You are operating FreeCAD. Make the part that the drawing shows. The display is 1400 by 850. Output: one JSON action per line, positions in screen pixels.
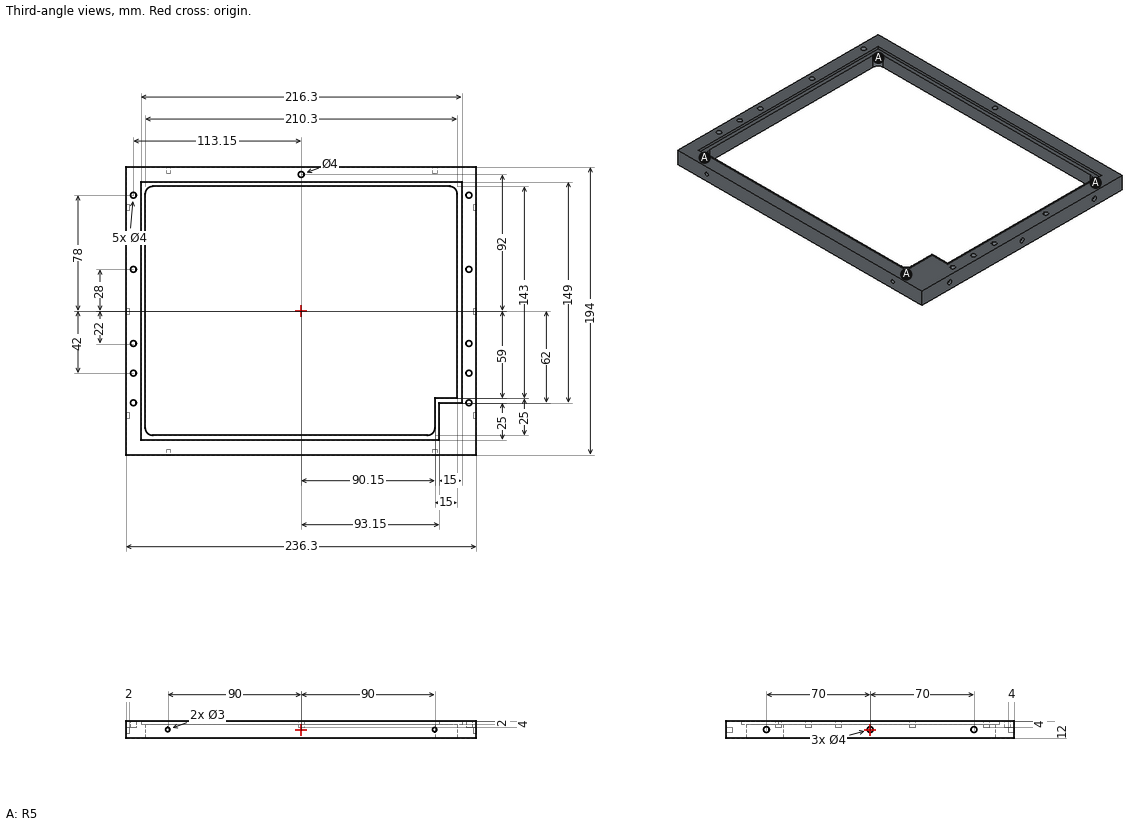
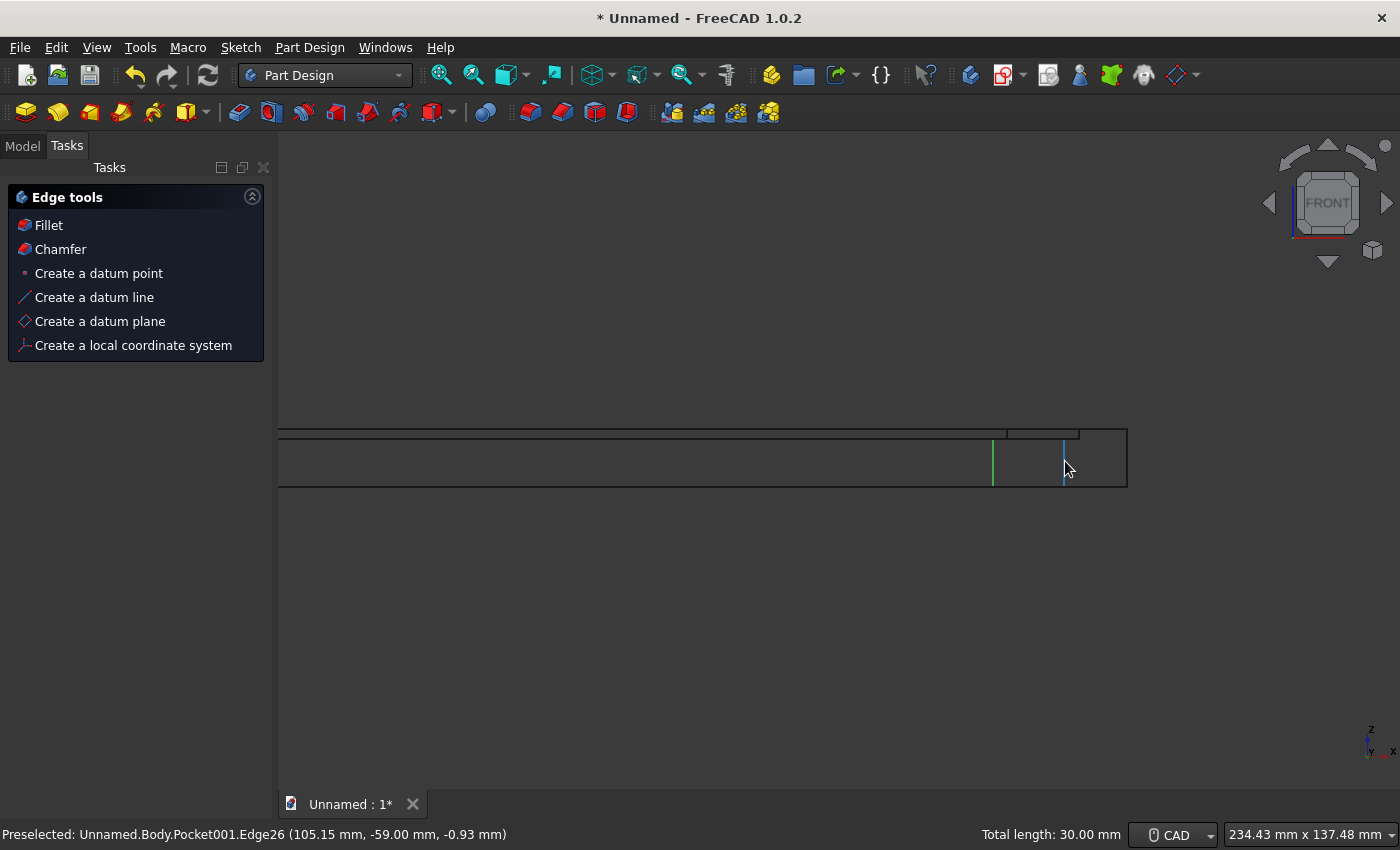
{"action": "left_click", "coordinate": [442, 76]}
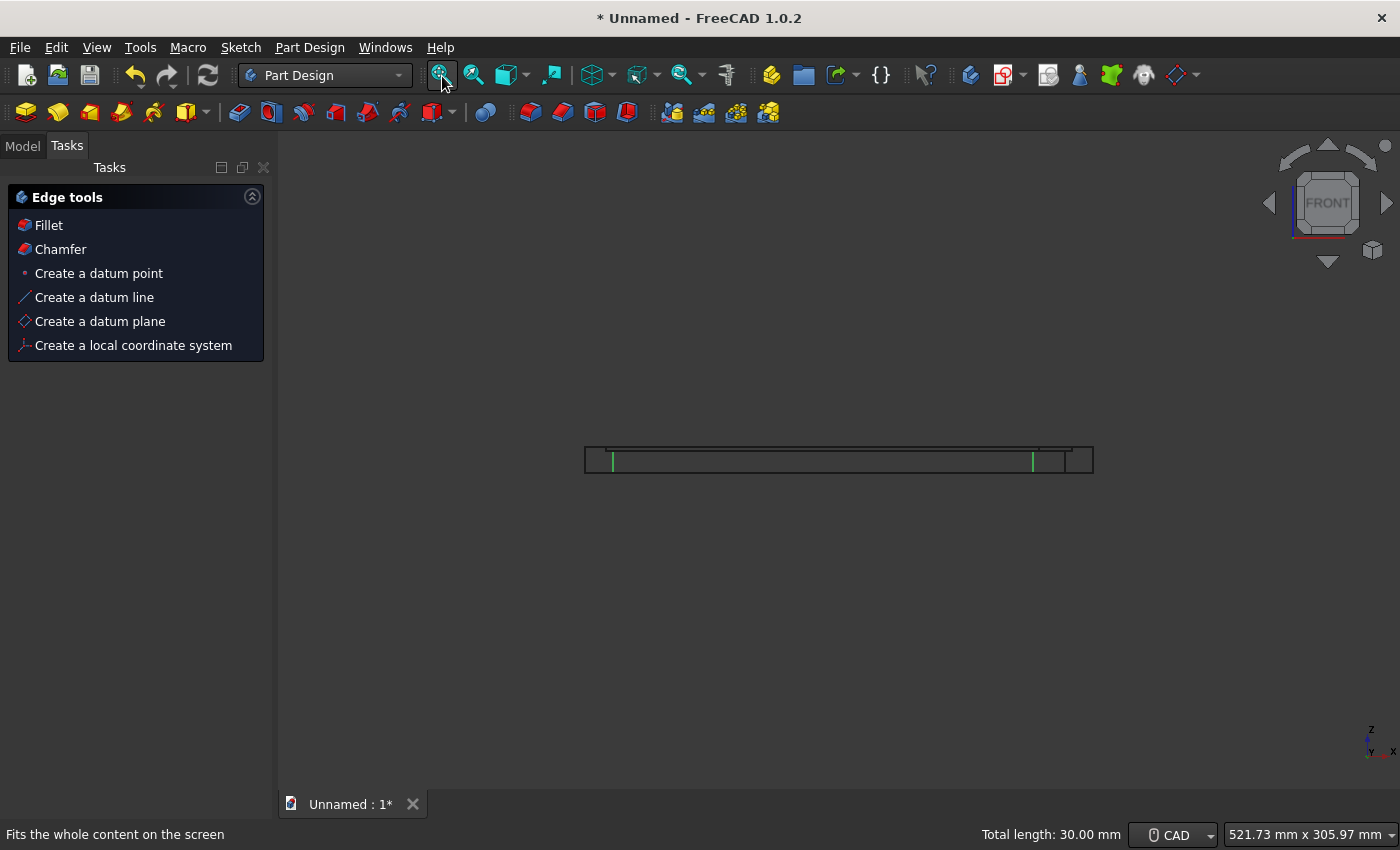
{"action": "key", "text": "3"}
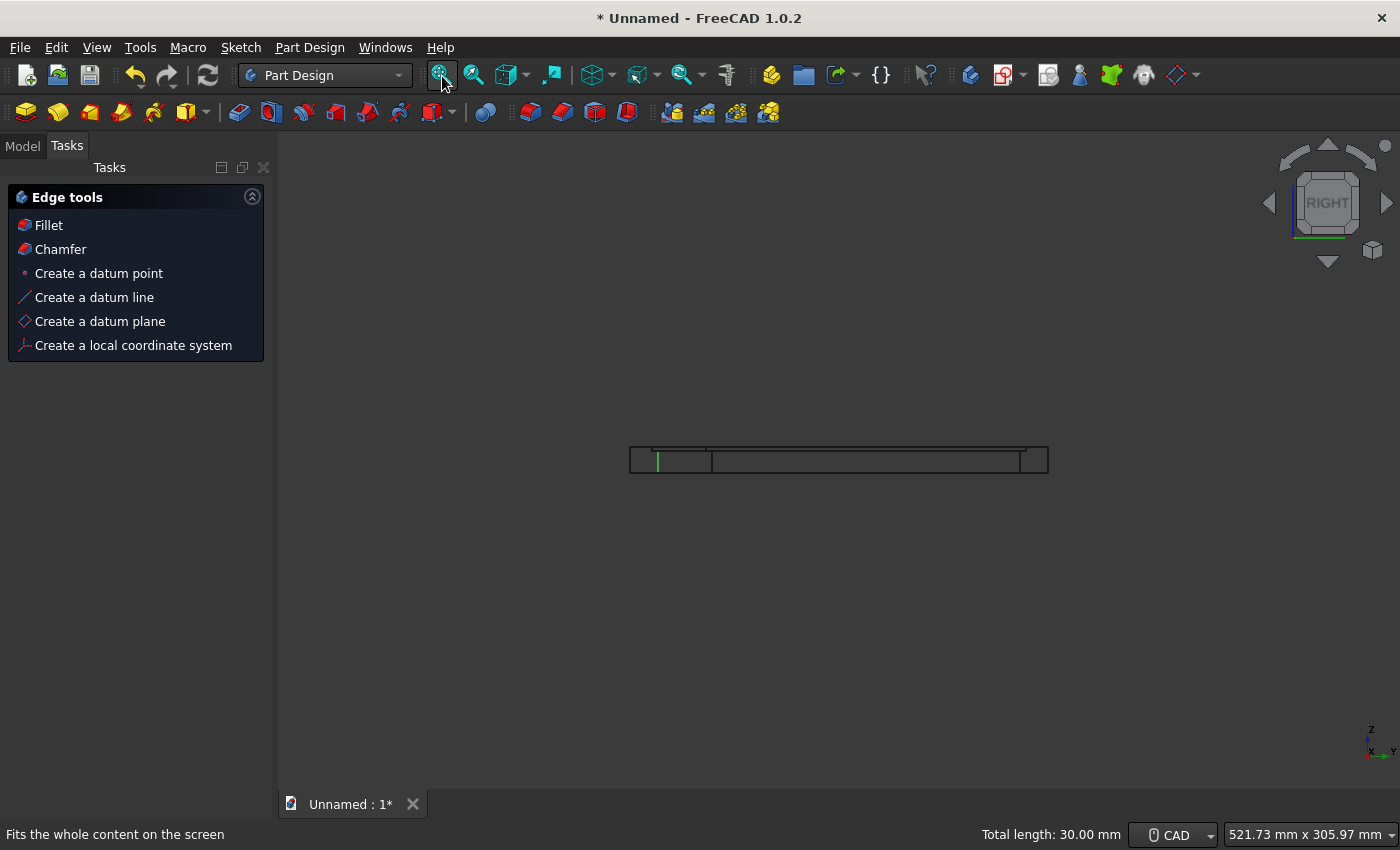
{"action": "left_click", "coordinate": [442, 76]}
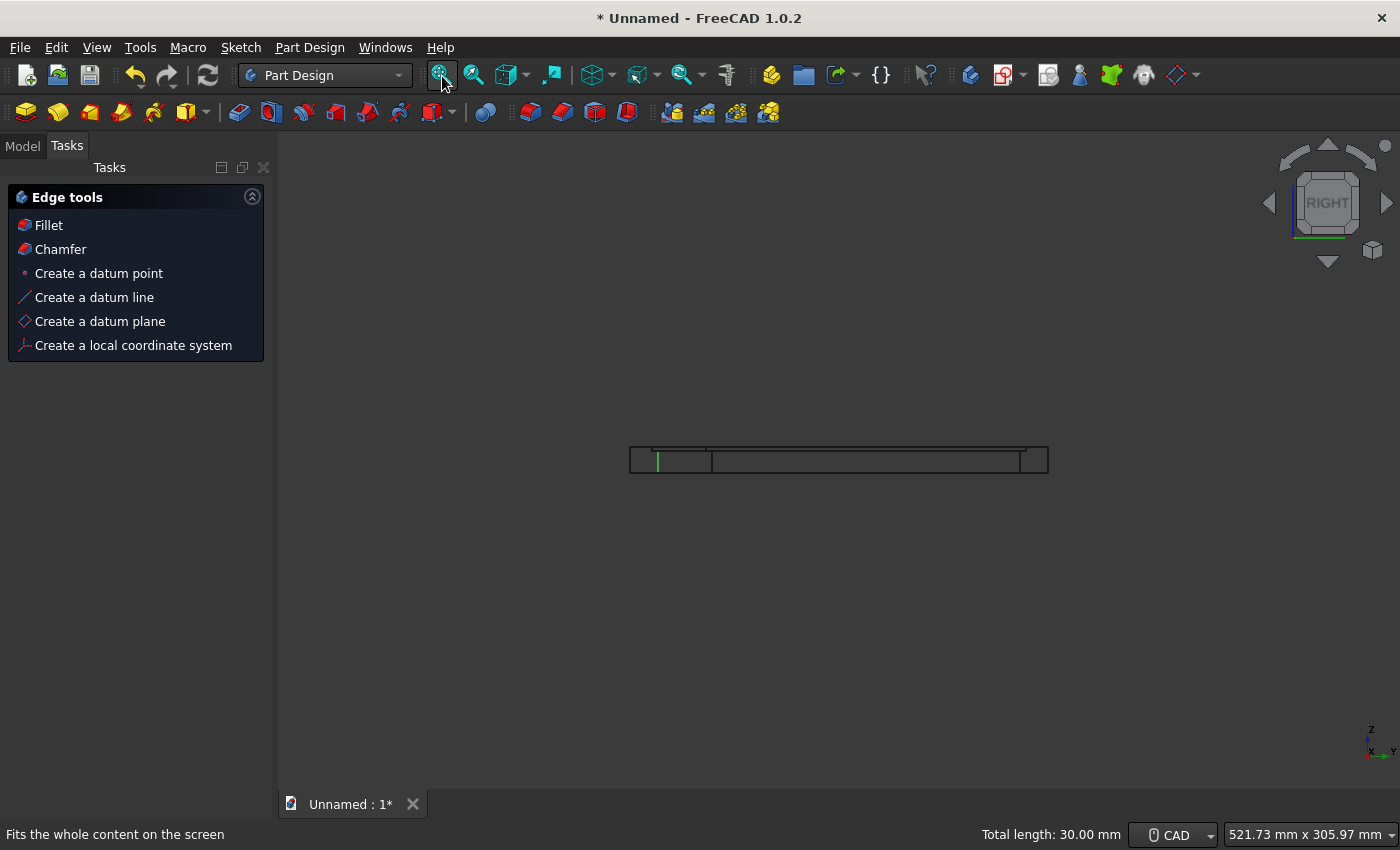
{"action": "left_click", "coordinate": [1020, 461], "text": "ctrl"}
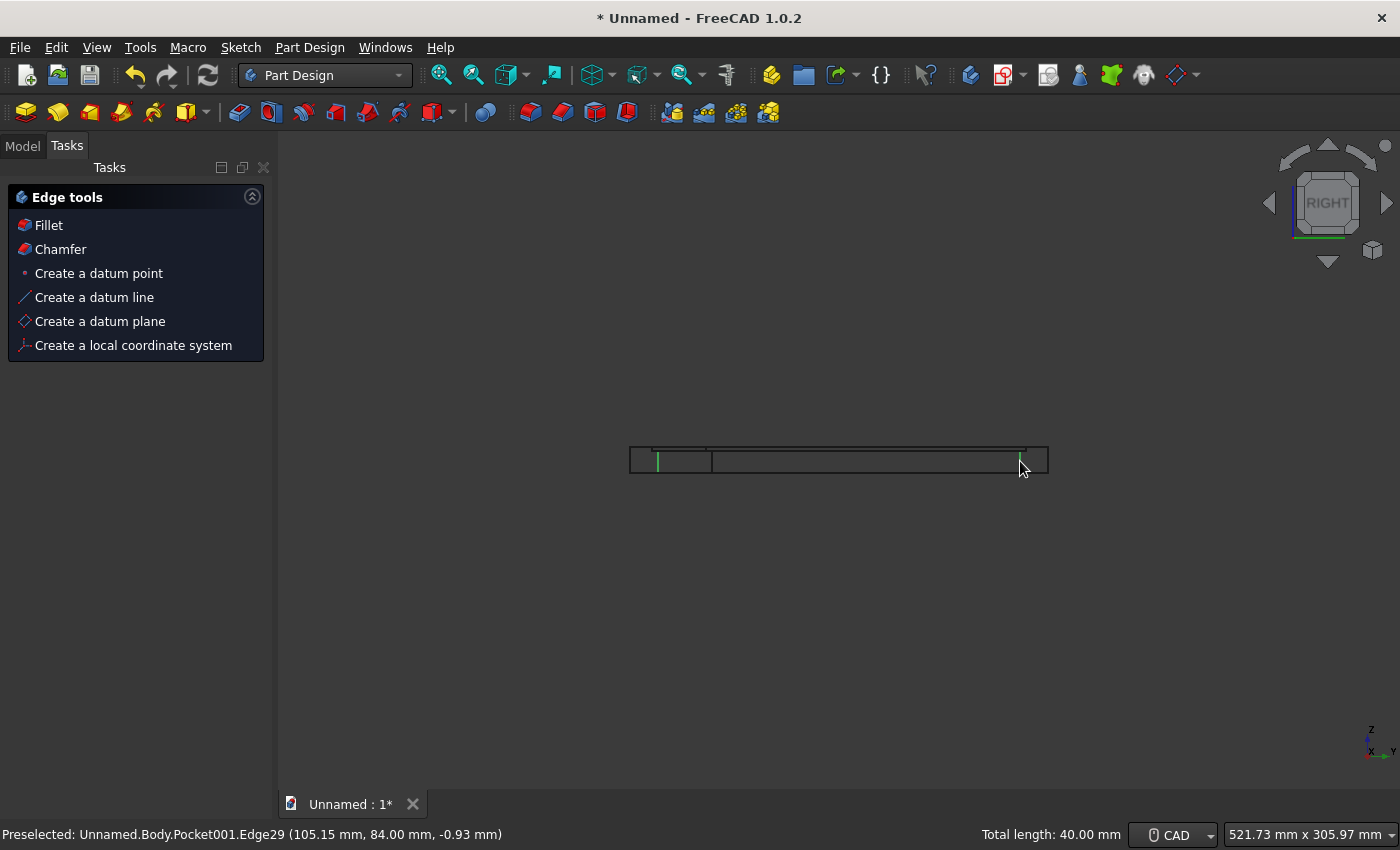
{"action": "key", "text": "v 1"}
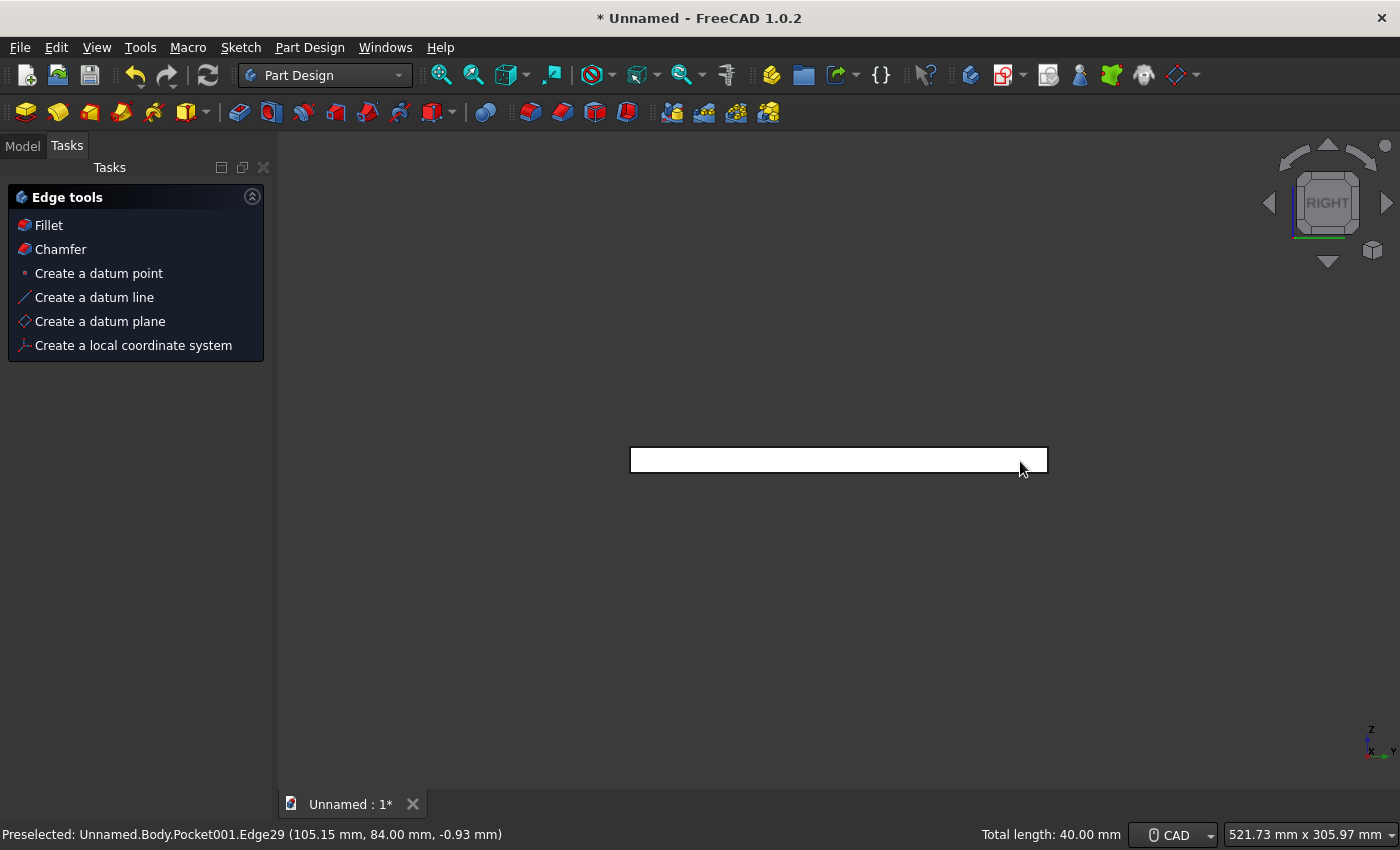
{"action": "left_click", "coordinate": [532, 112]}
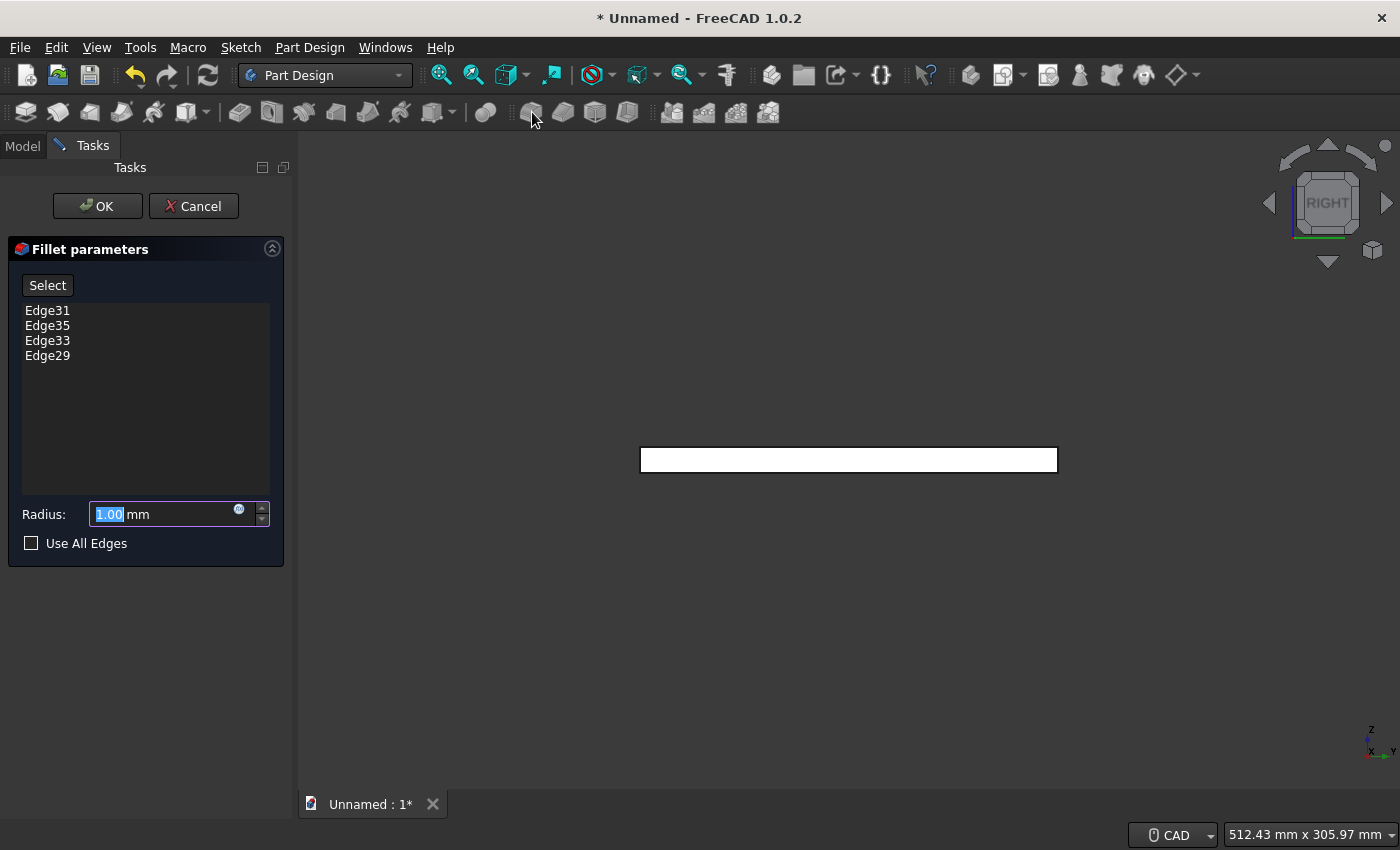
{"action": "type", "text": "5"}
{"action": "key", "text": "Tab"}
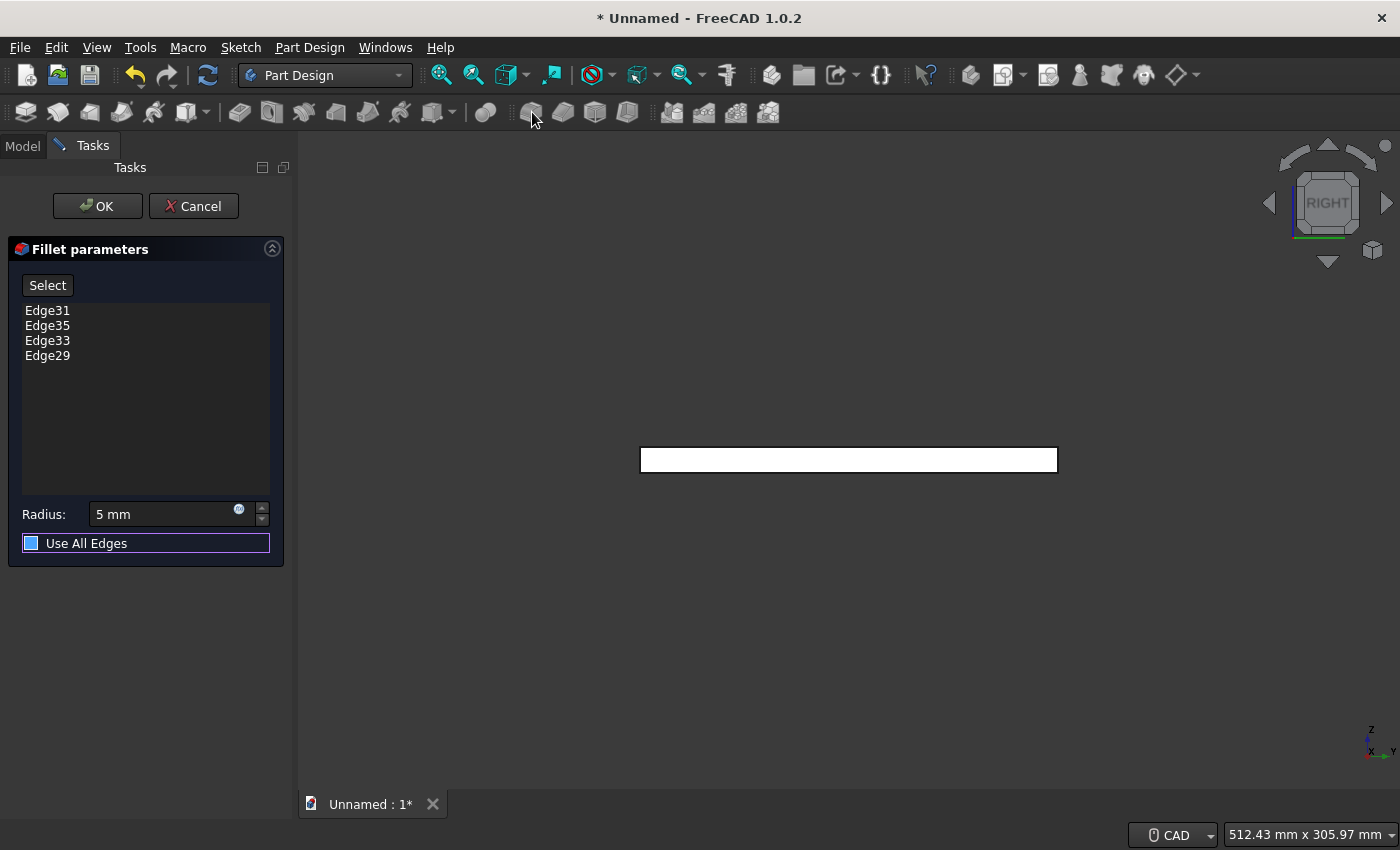
{"action": "left_click", "coordinate": [98, 206]}